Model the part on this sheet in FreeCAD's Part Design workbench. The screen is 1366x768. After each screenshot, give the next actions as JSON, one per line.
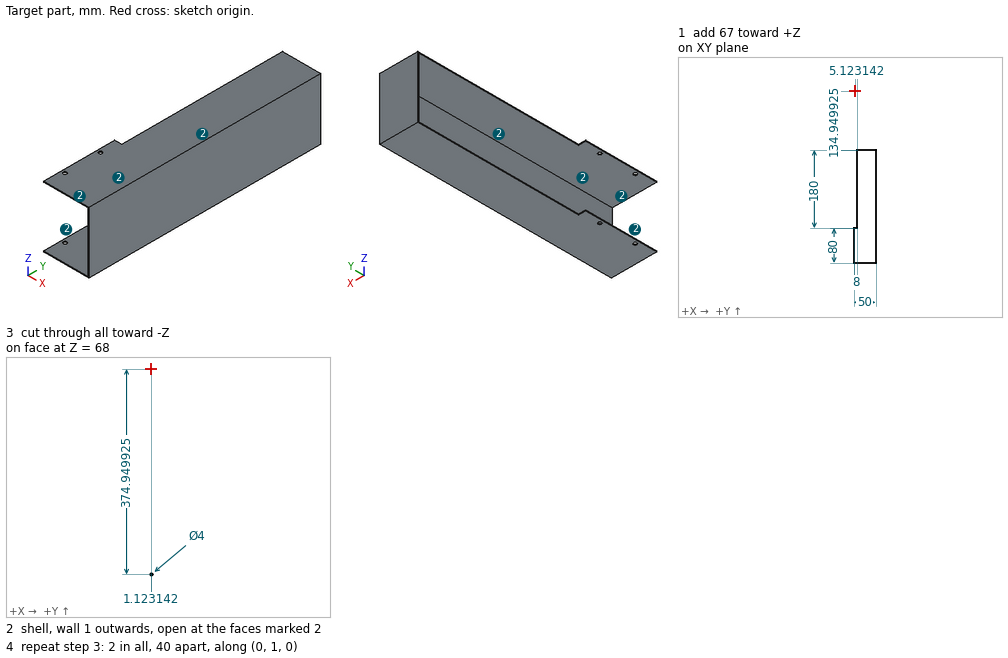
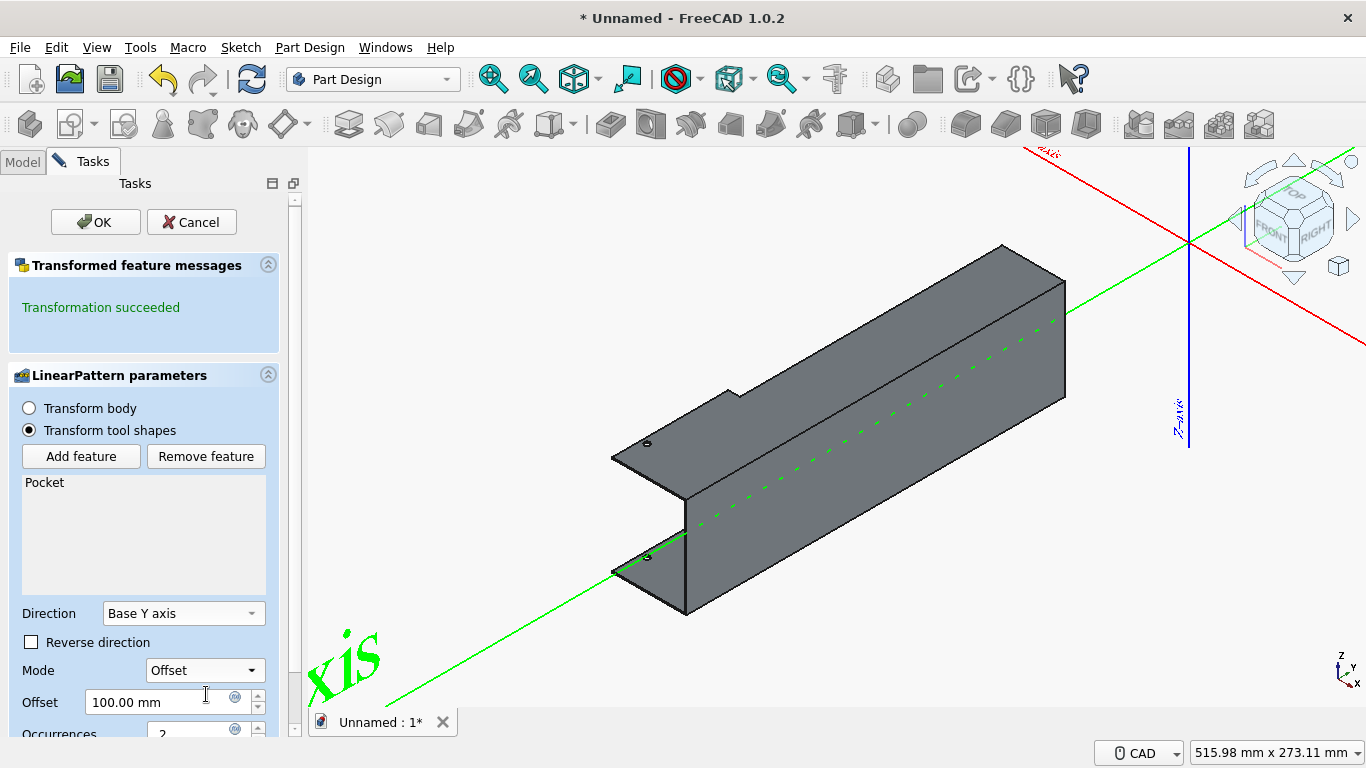
{"action": "triple_click", "coordinate": [168, 702]}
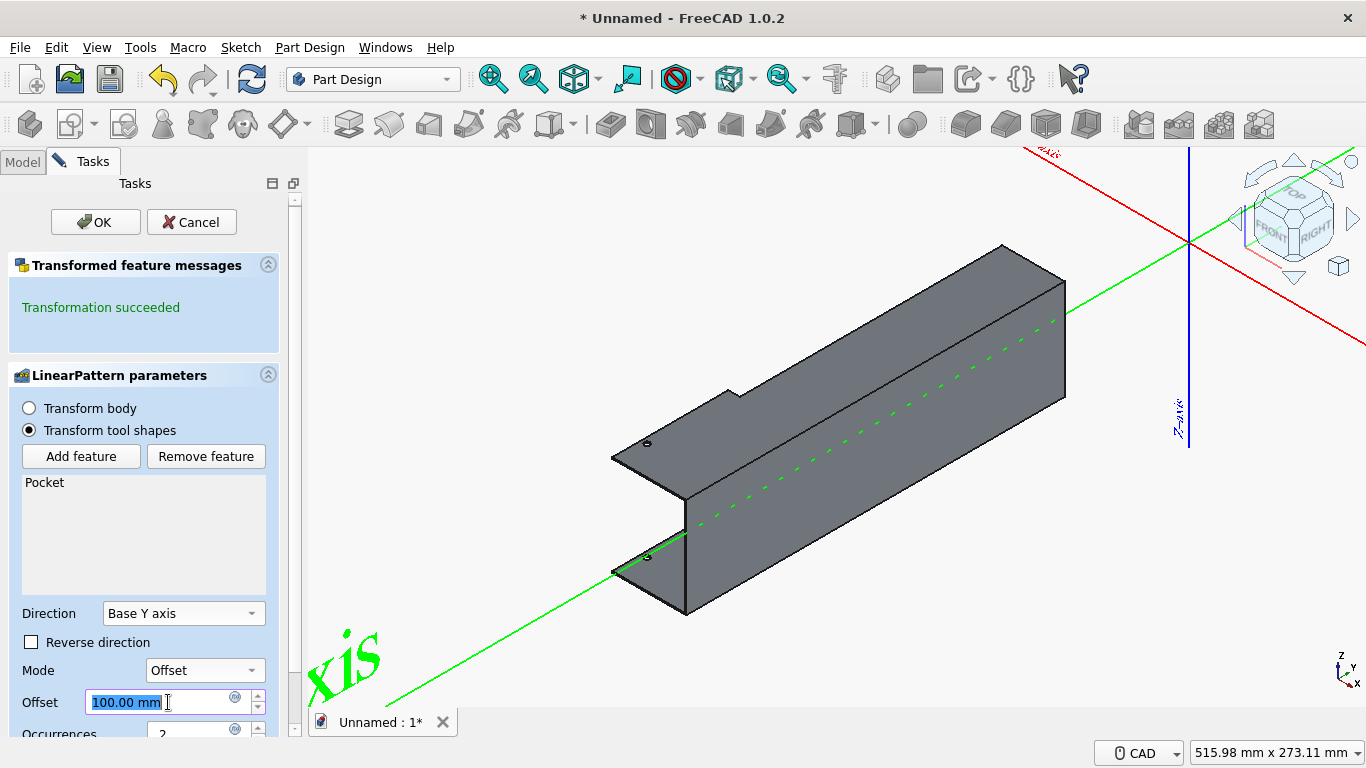
{"action": "type", "text": "40"}
{"action": "key", "text": "Tab"}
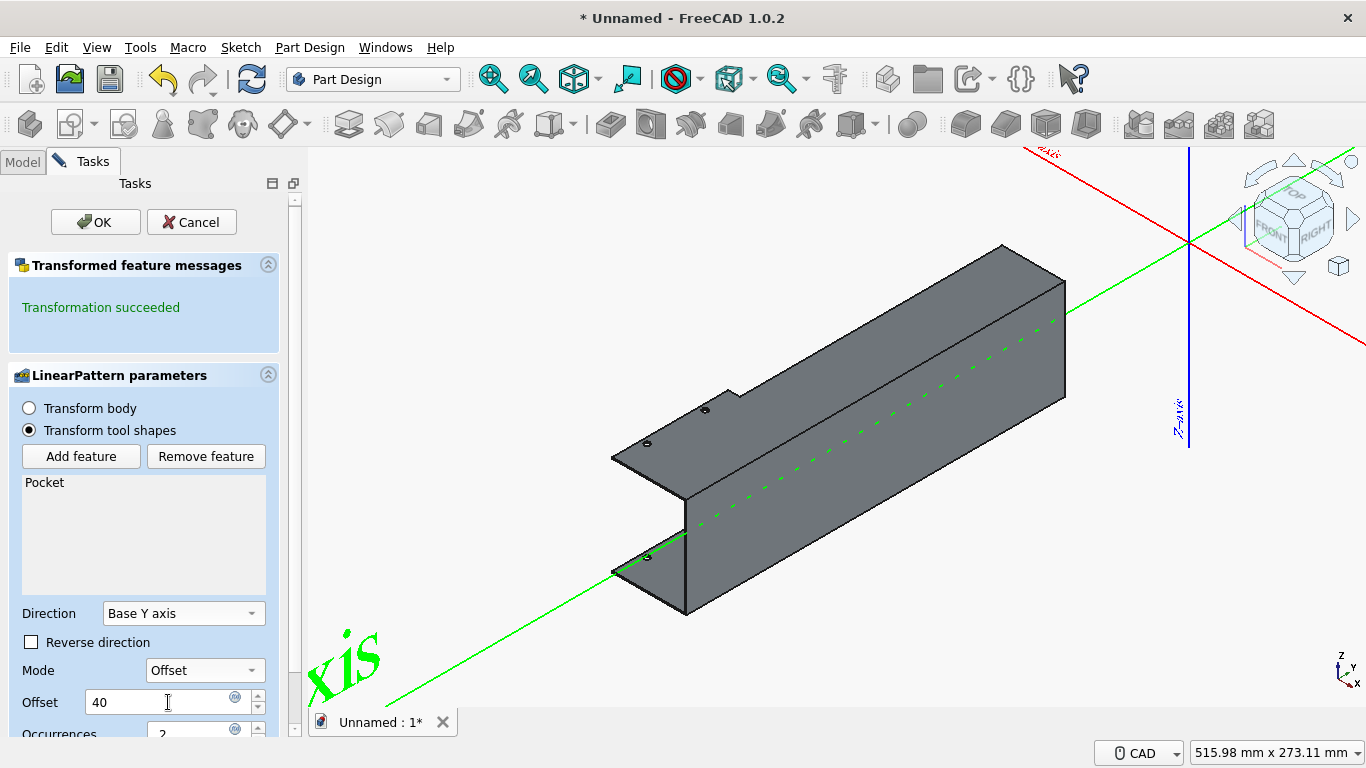
{"action": "scroll", "coordinate": [295, 464], "scroll_direction": "down", "scroll_amount": 2}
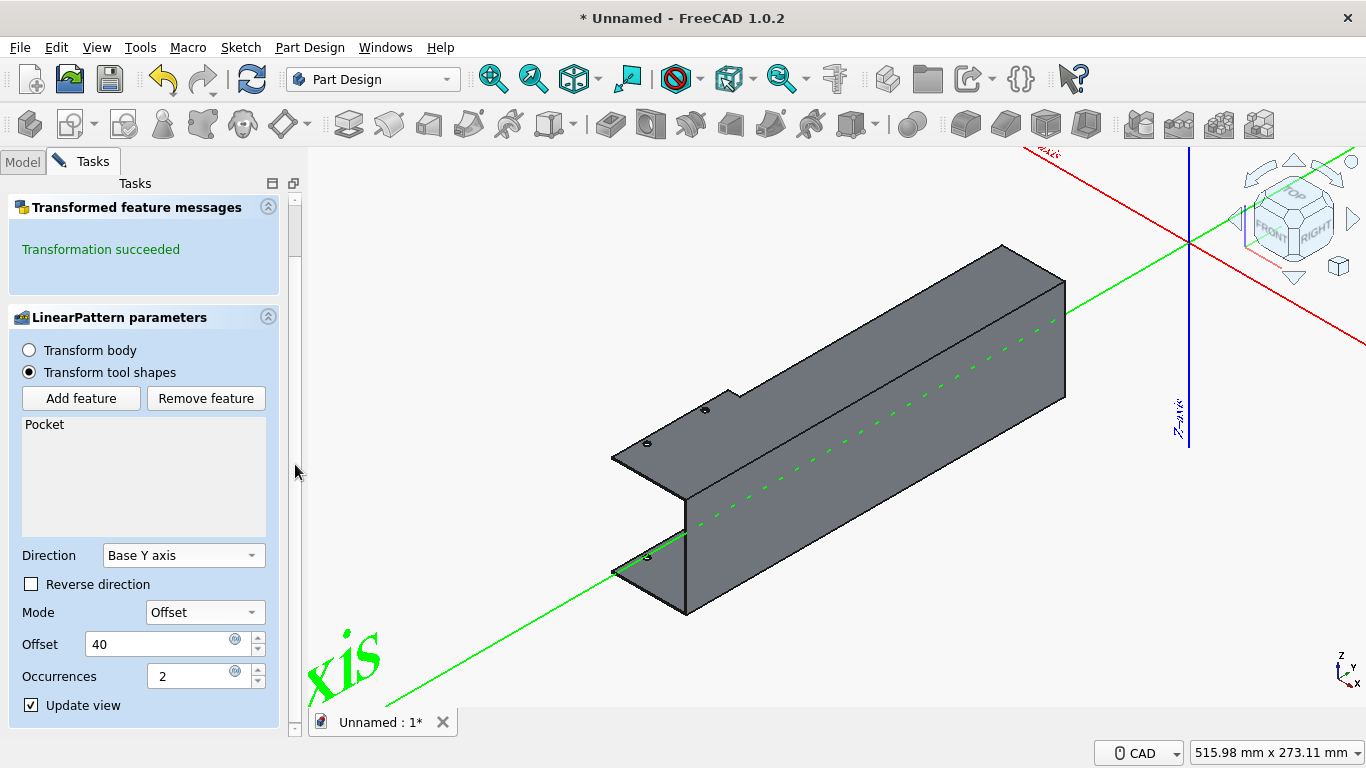
{"action": "triple_click", "coordinate": [198, 676]}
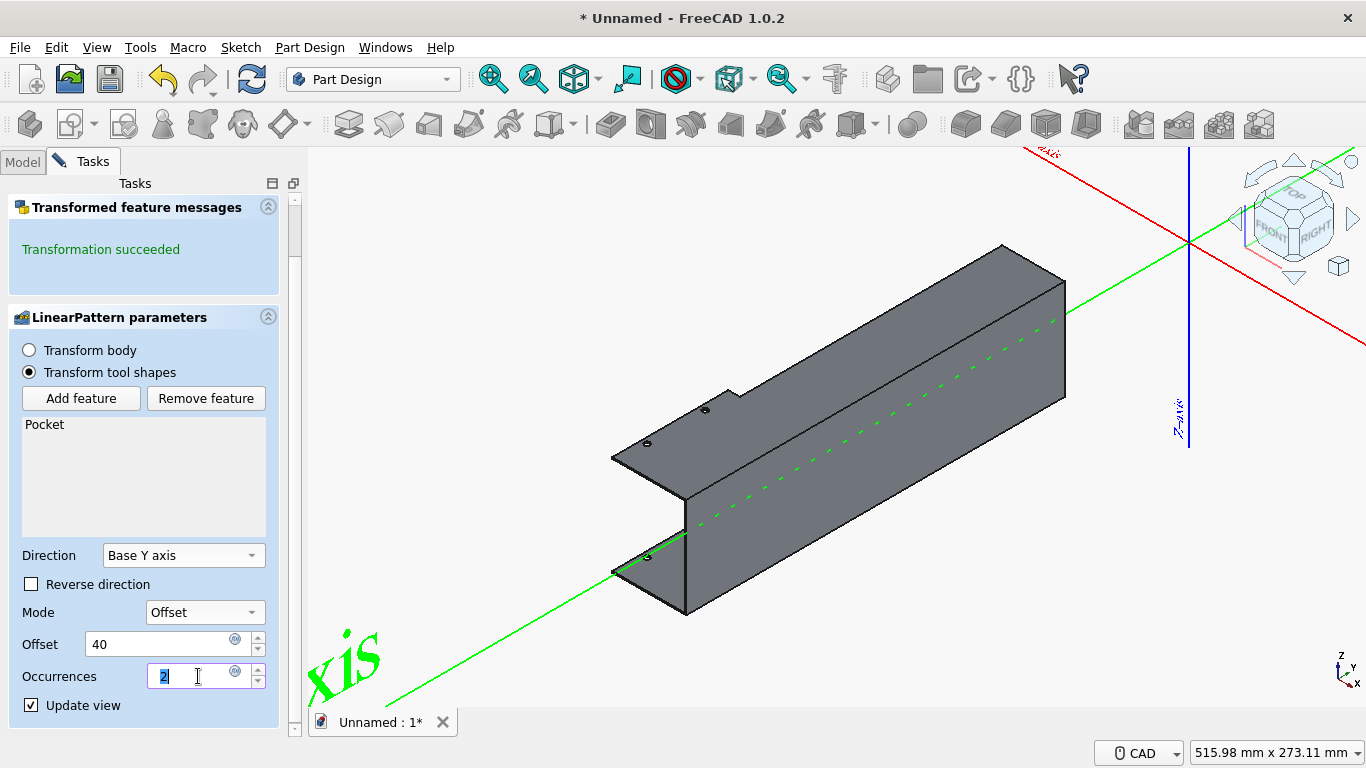
{"action": "type", "text": "2"}
{"action": "key", "text": "Tab"}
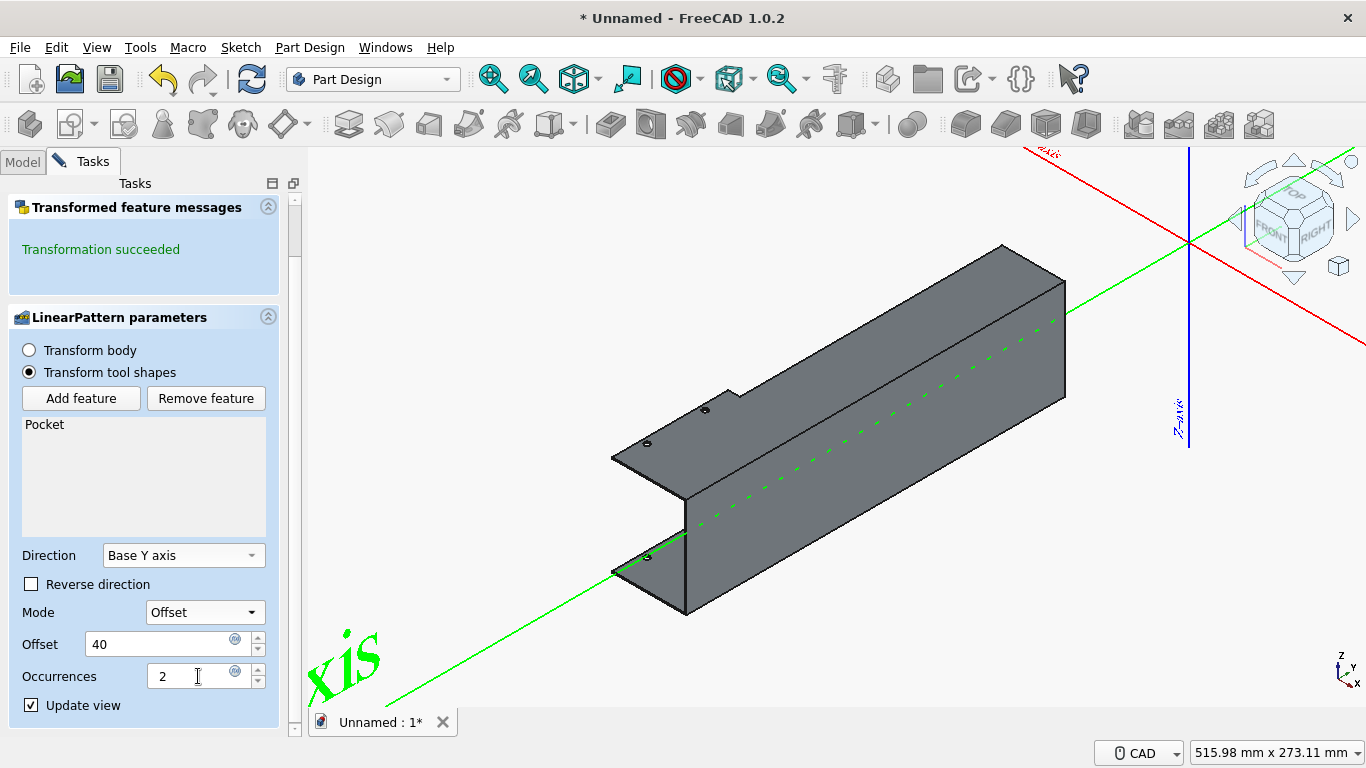
{"action": "scroll", "coordinate": [295, 464], "scroll_direction": "up", "scroll_amount": 2}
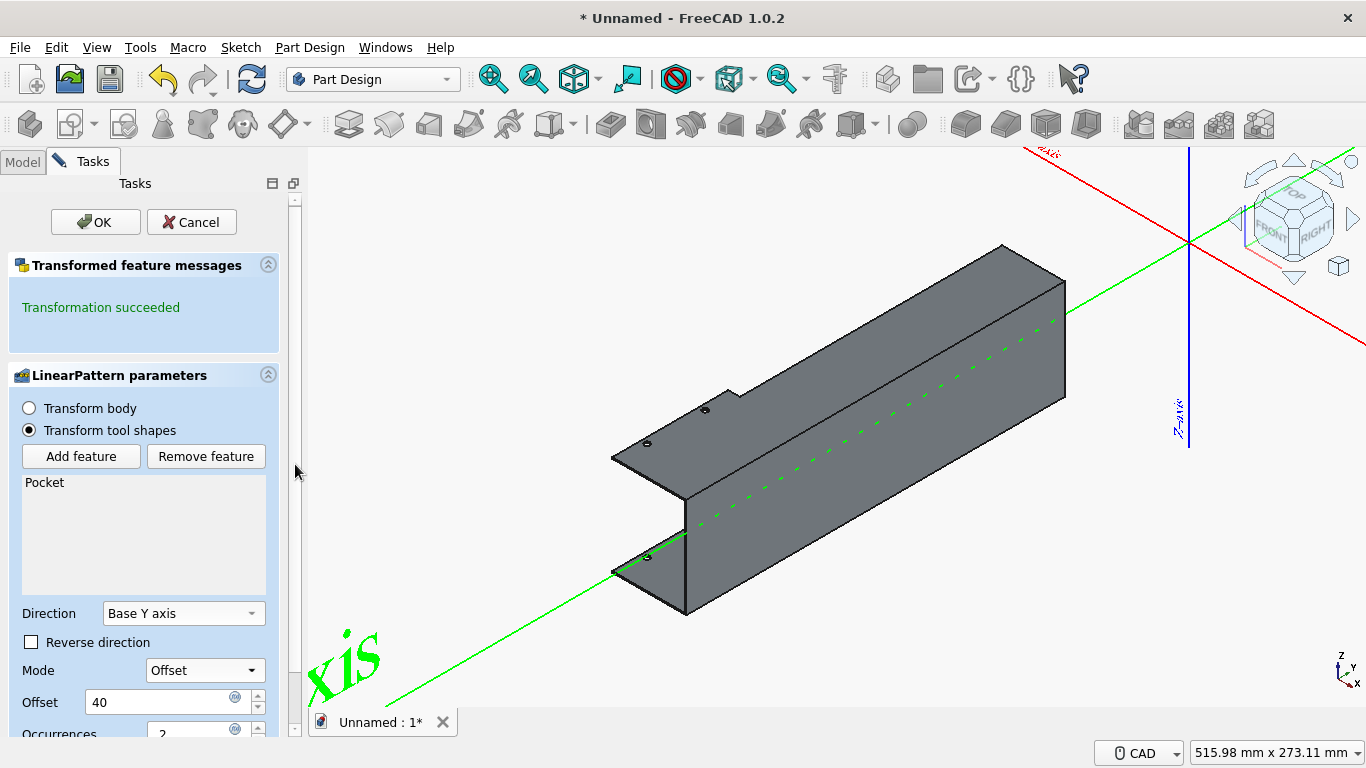
{"action": "left_click", "coordinate": [96, 222]}